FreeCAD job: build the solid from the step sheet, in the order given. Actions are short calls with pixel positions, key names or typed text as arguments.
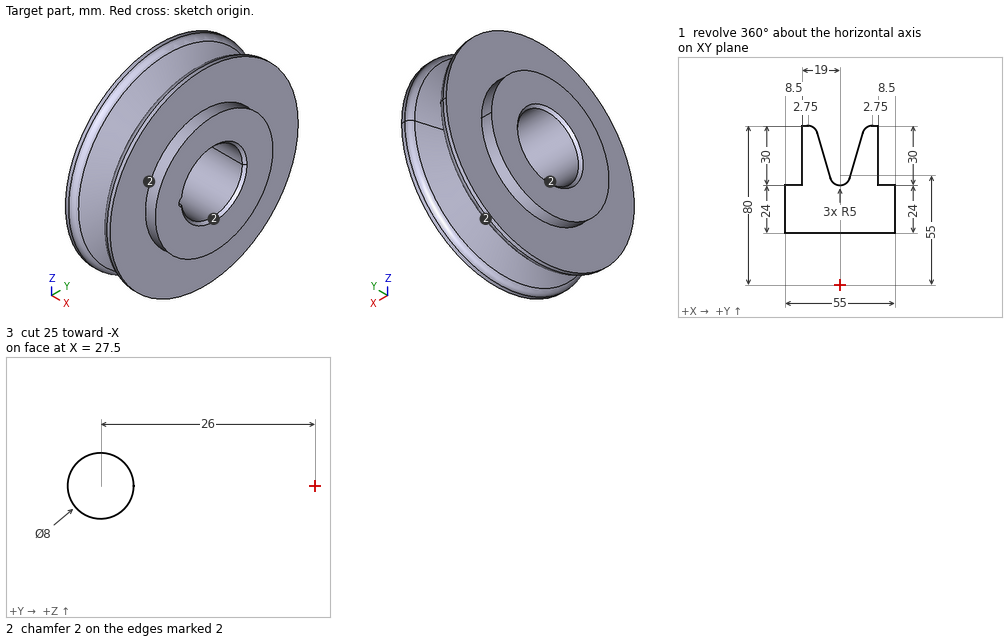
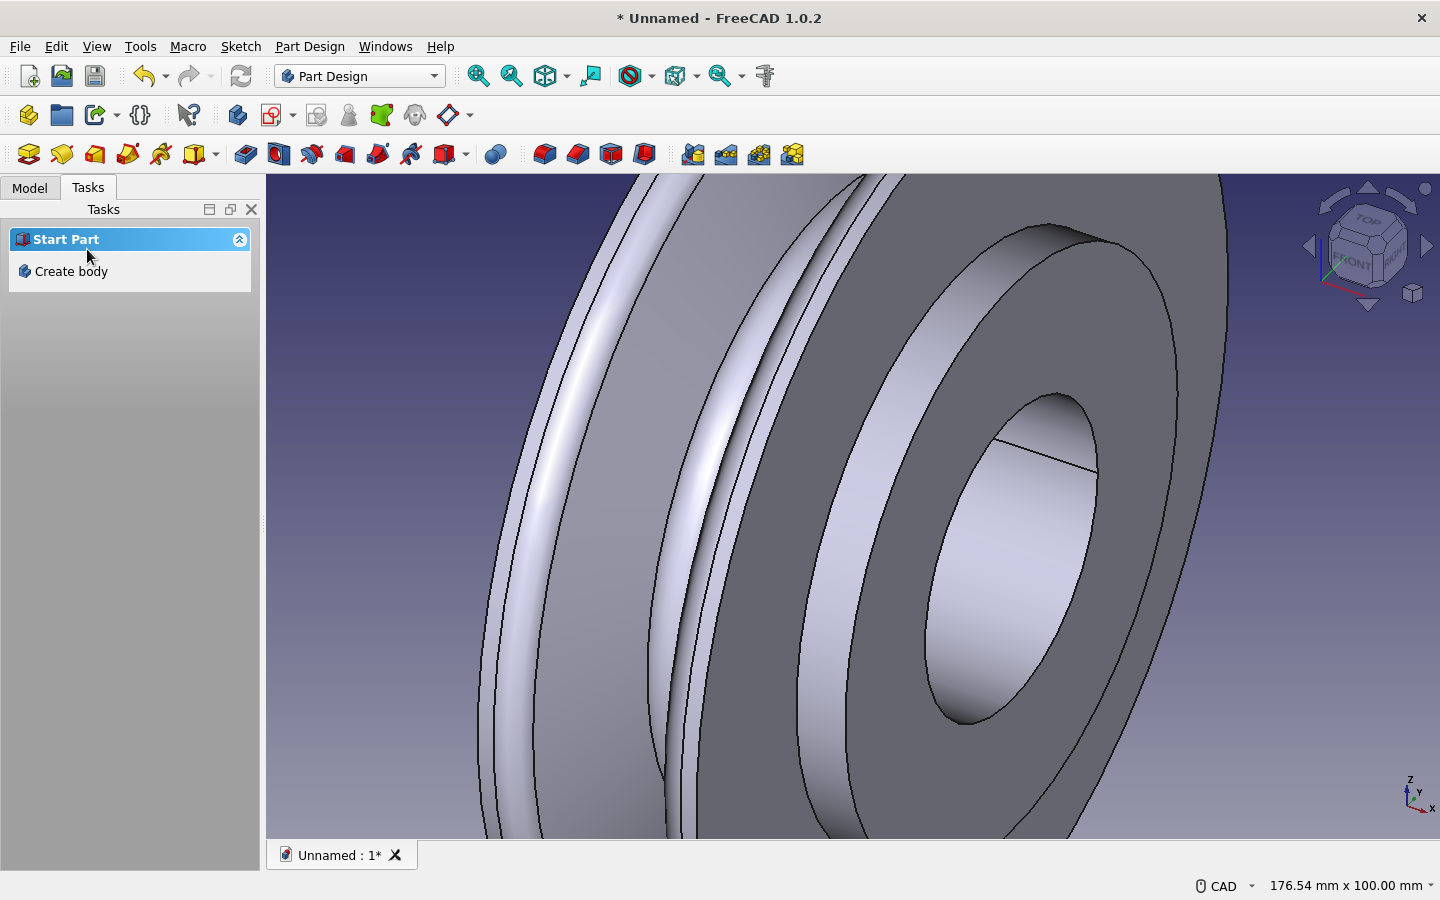
key(v)
key(f)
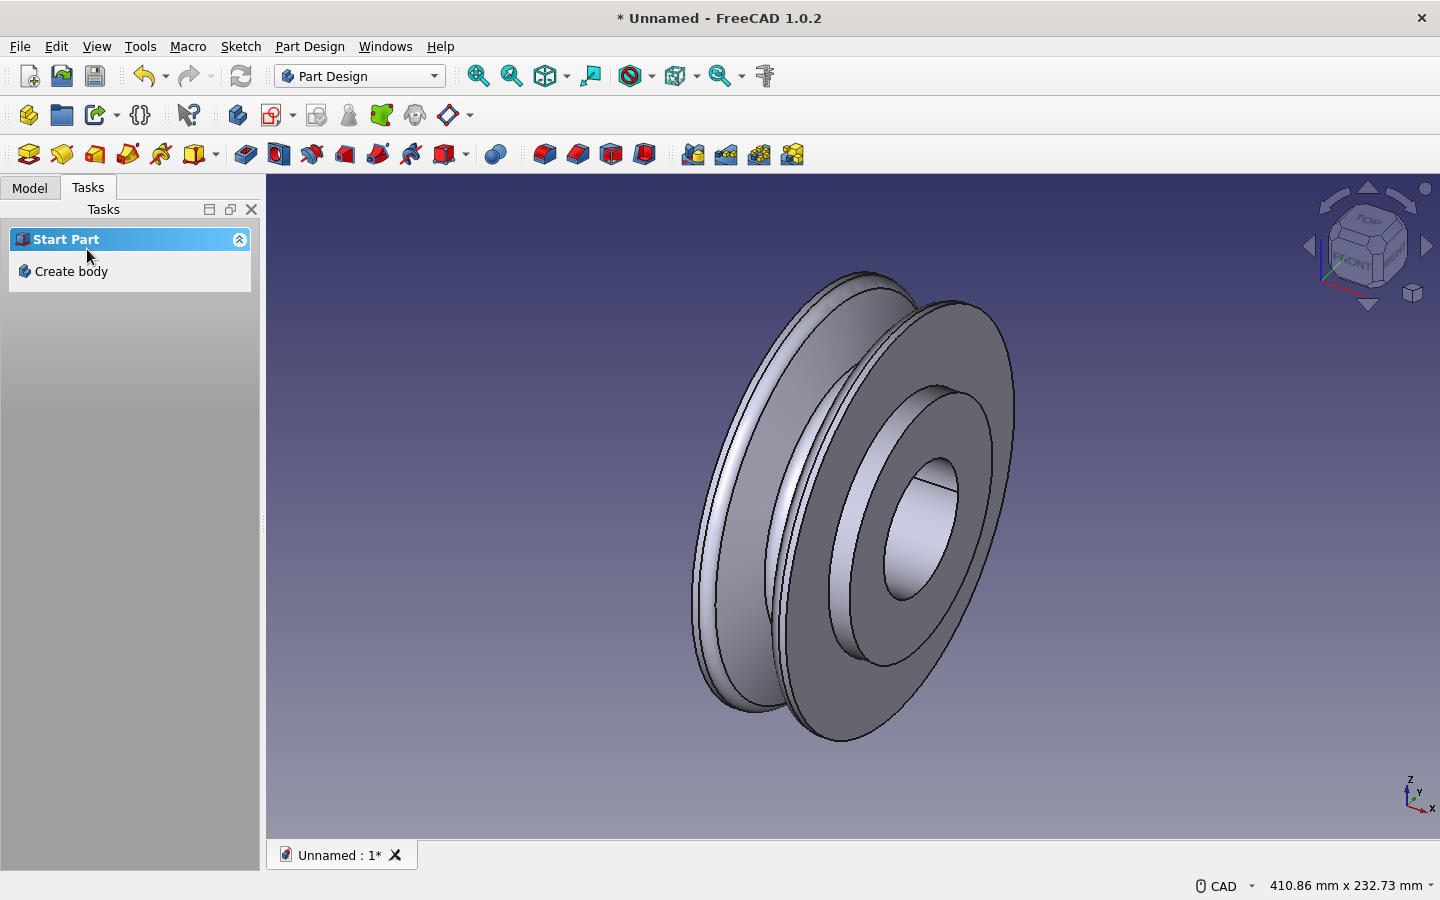
click(909, 597)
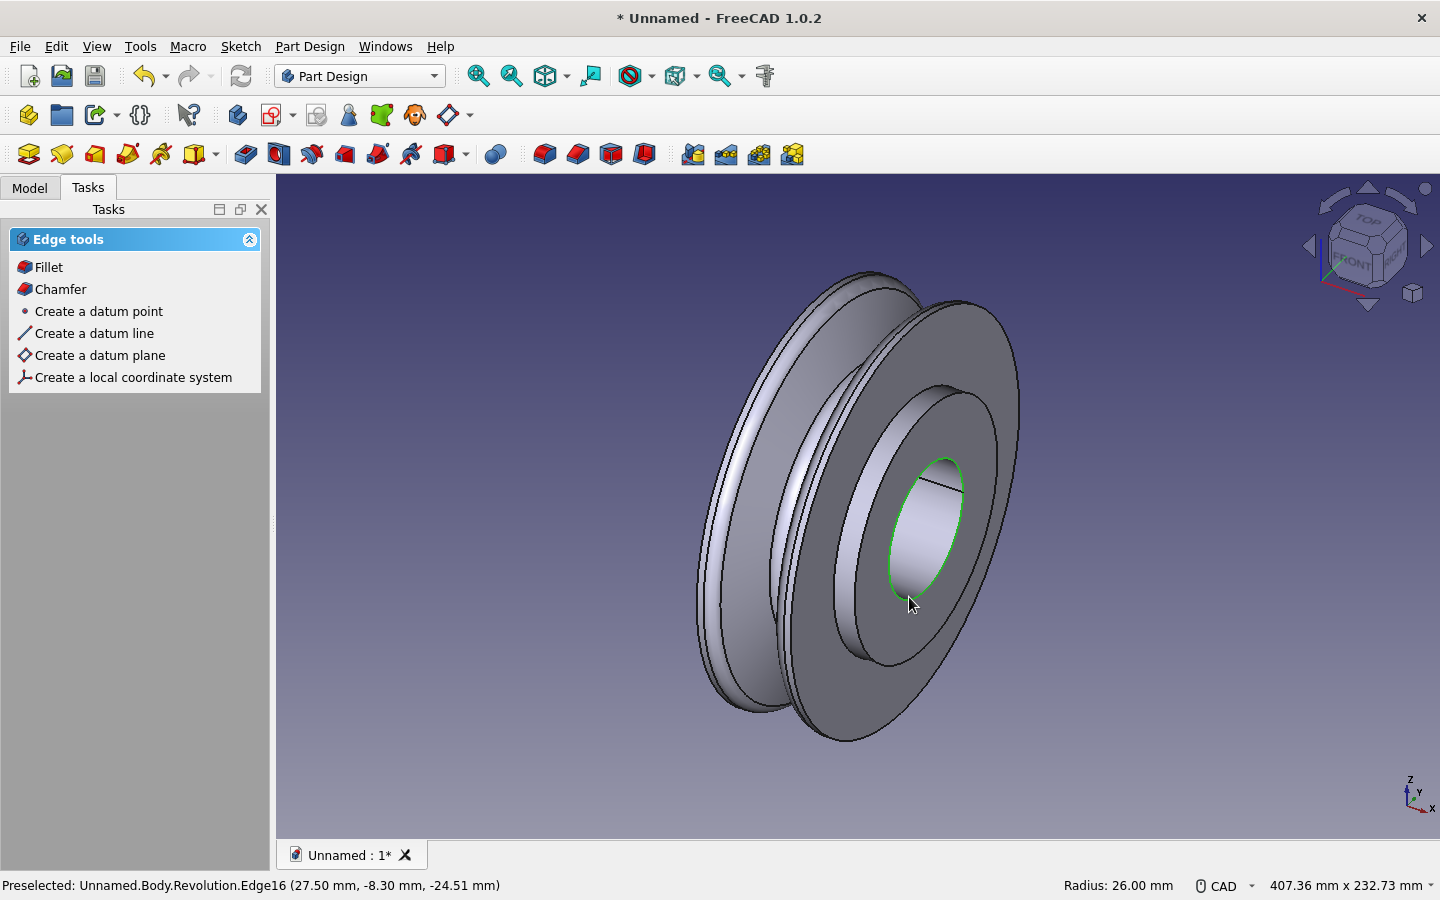
key(0)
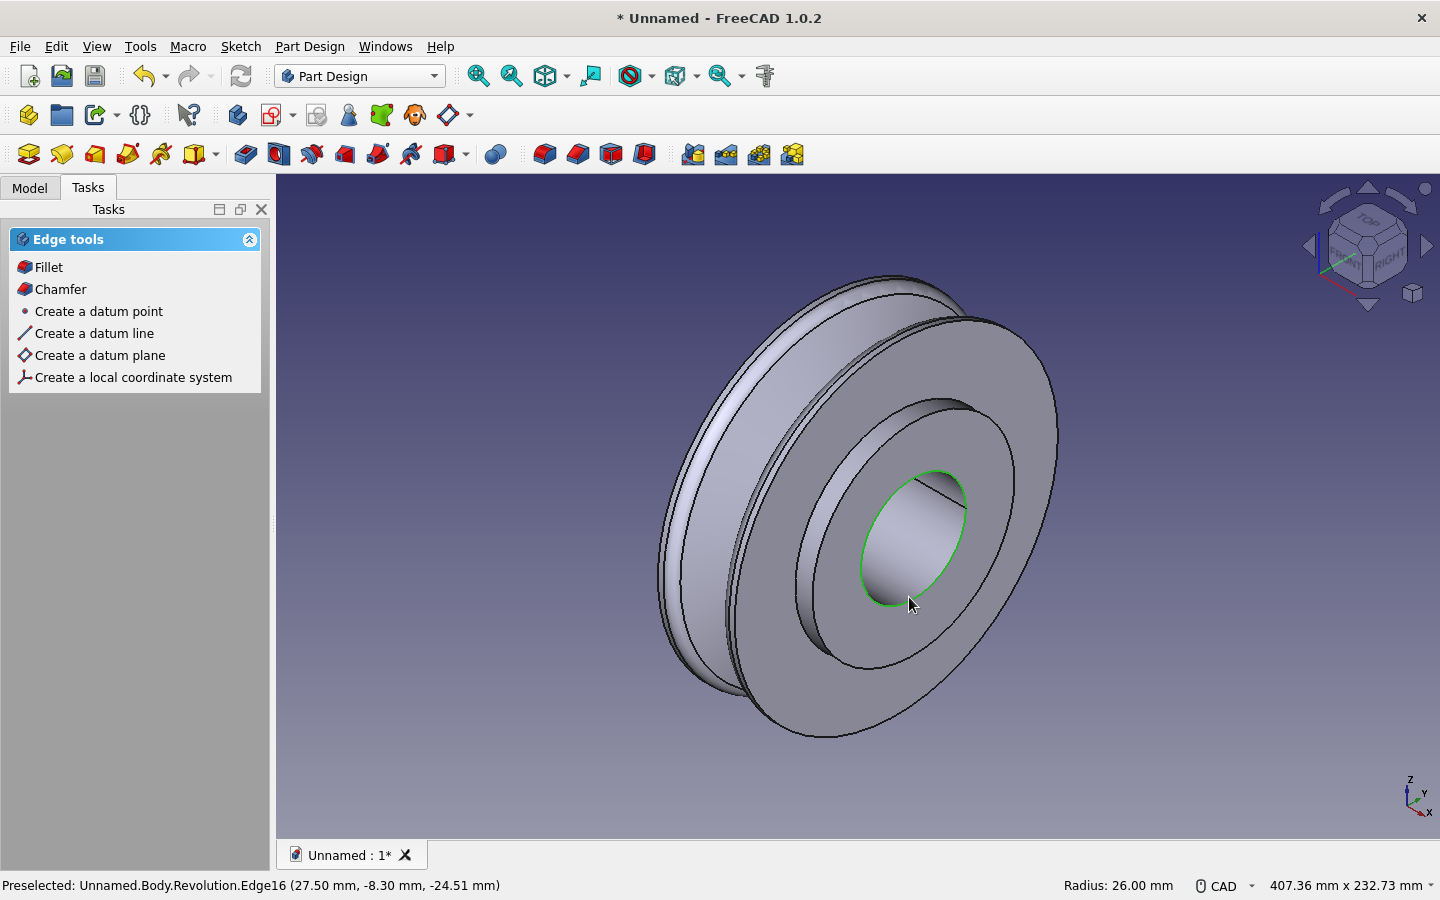
key(2)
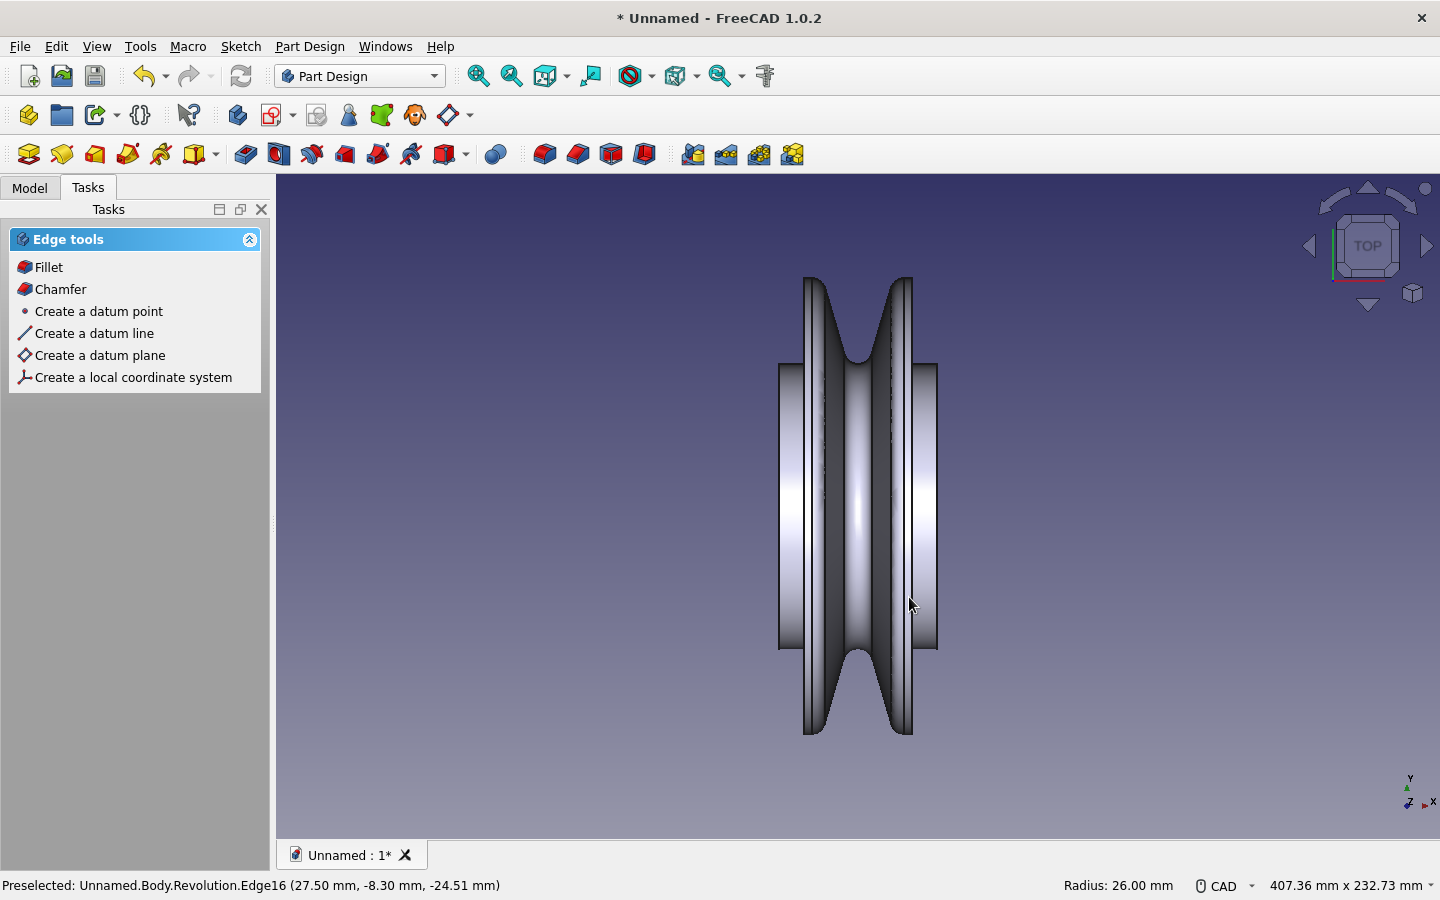
key(1)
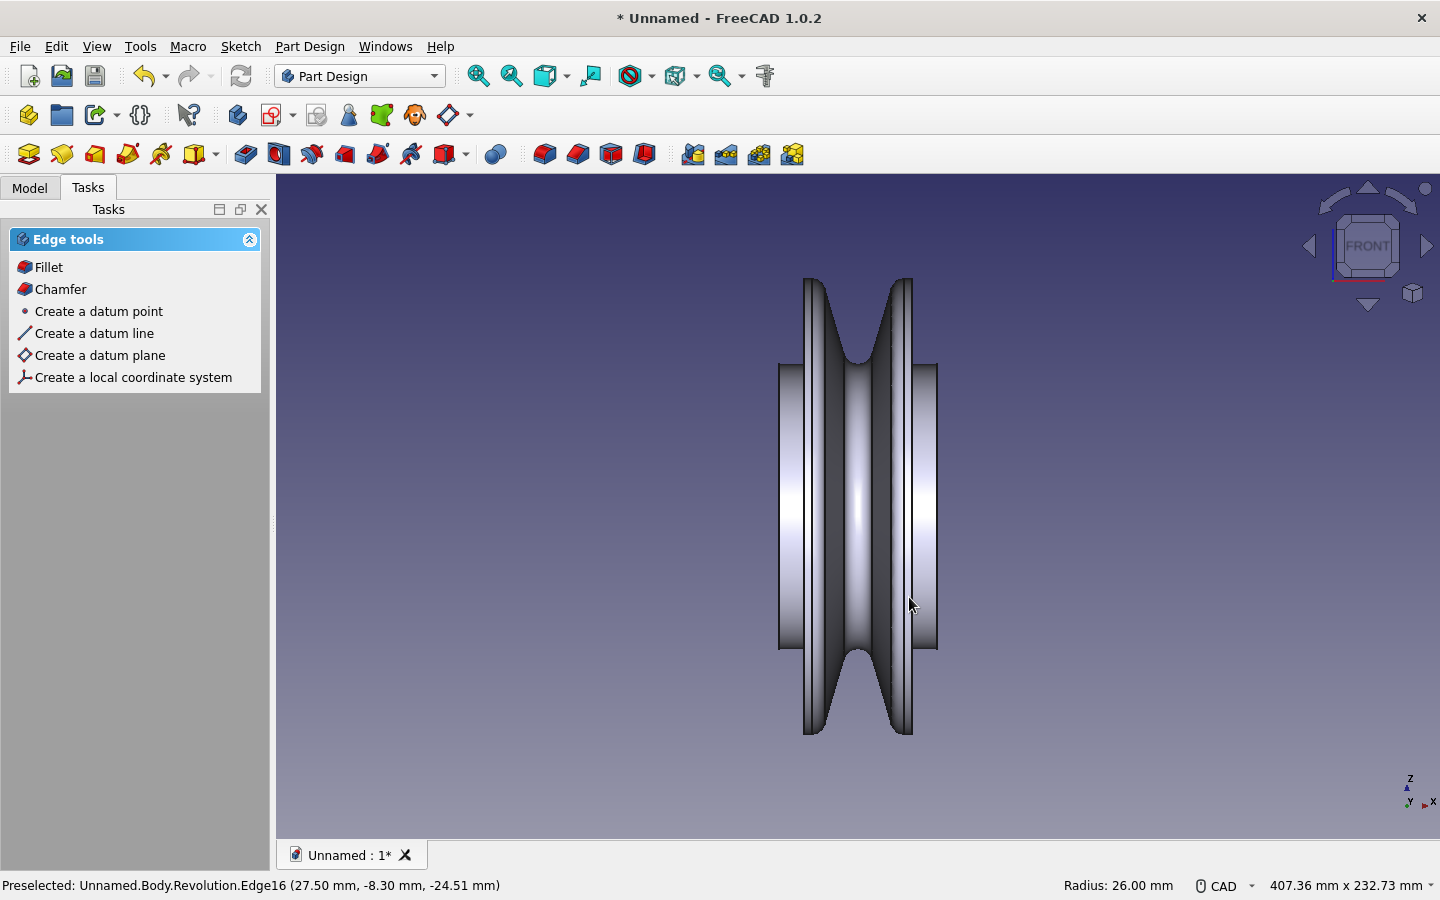
key(3)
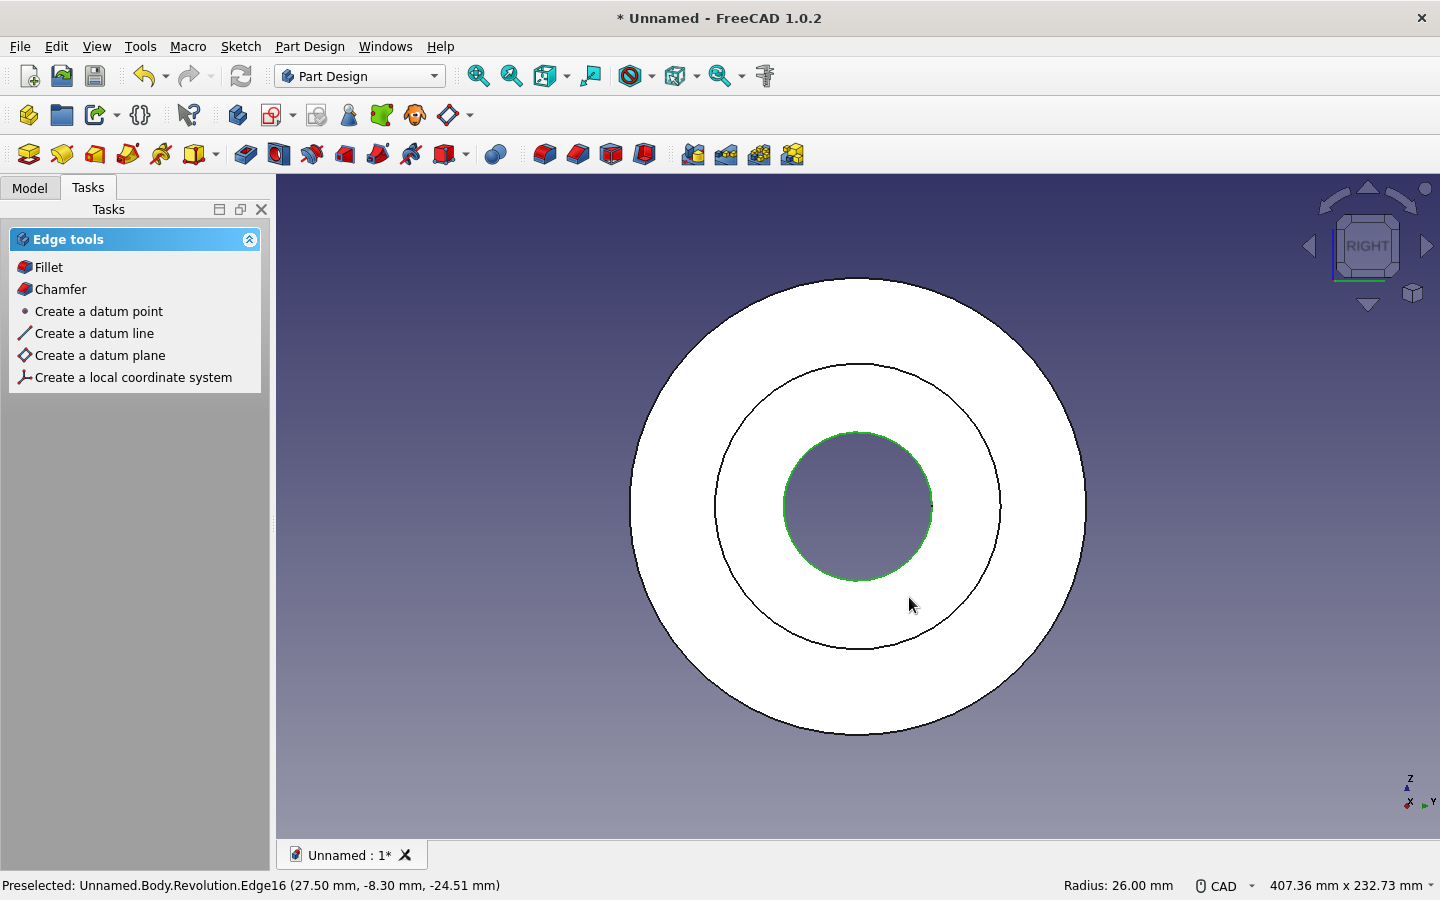
key(5)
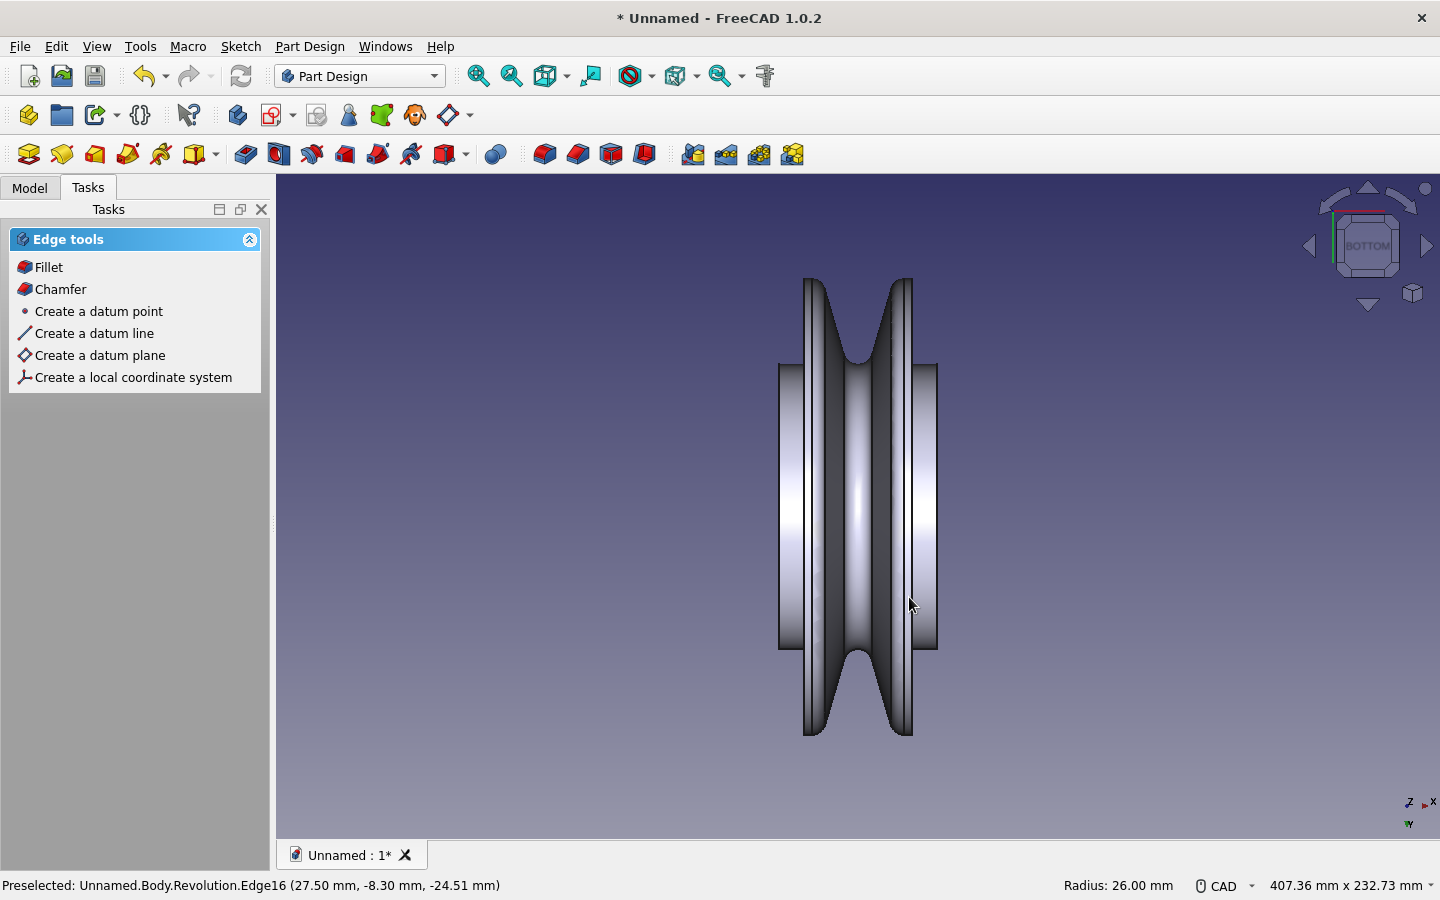
key(4)